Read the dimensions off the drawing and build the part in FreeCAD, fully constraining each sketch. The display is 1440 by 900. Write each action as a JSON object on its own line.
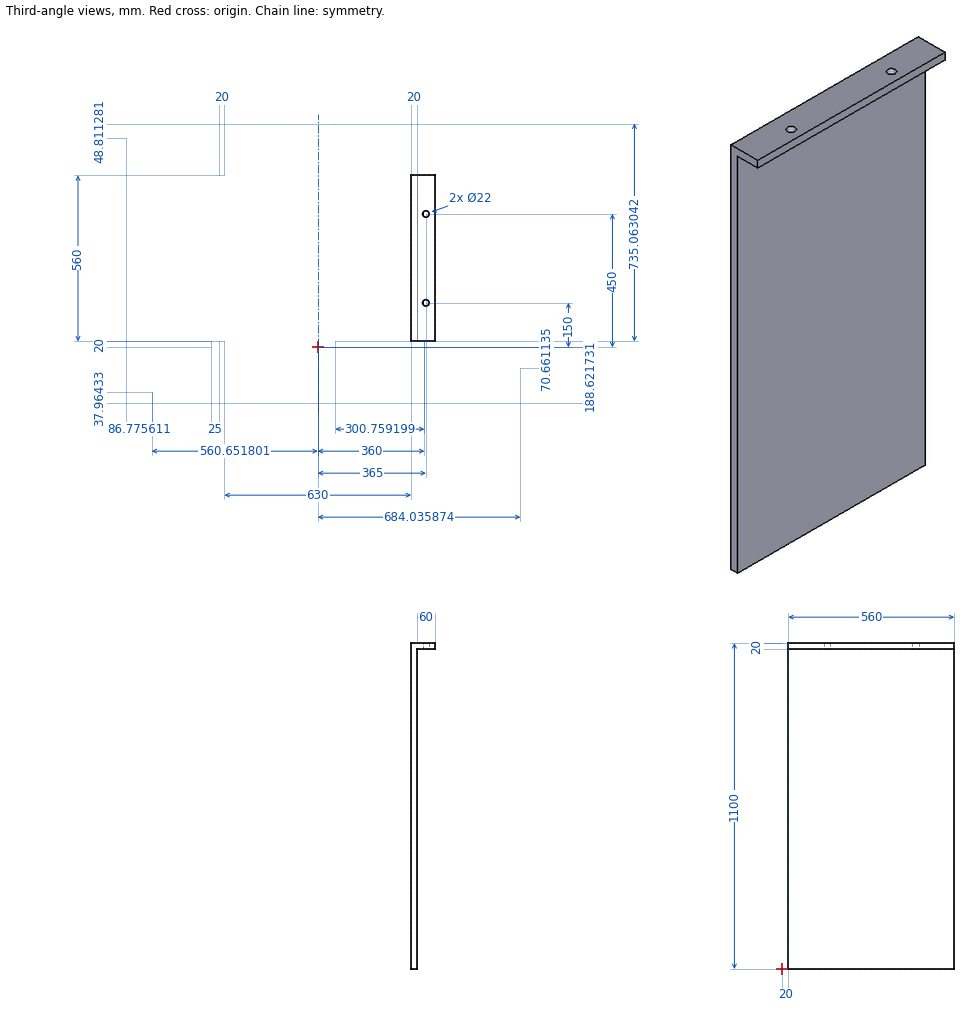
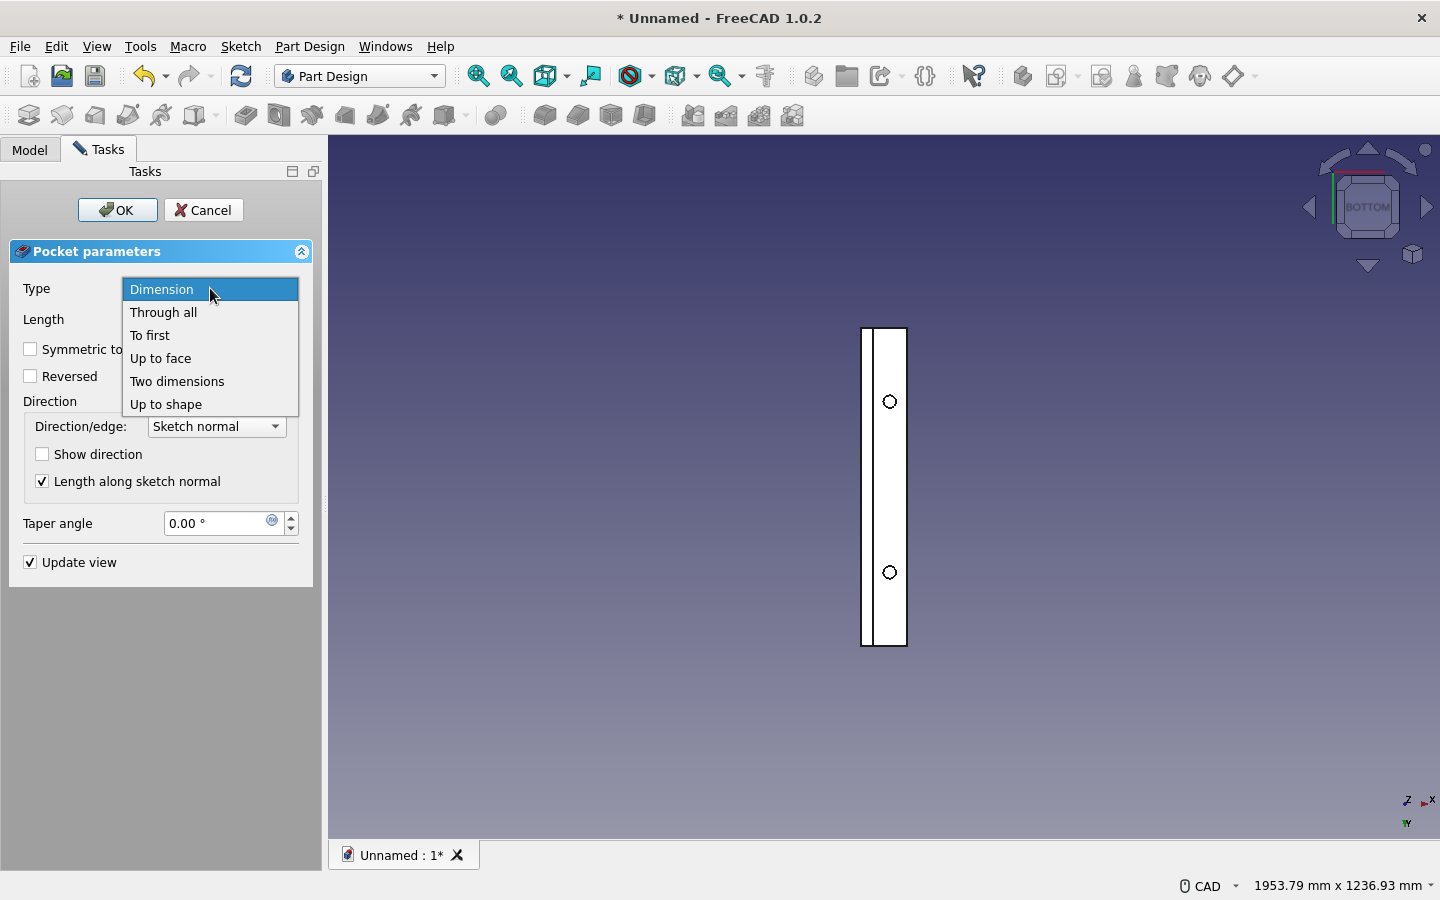
{"action": "left_click", "coordinate": [208, 312]}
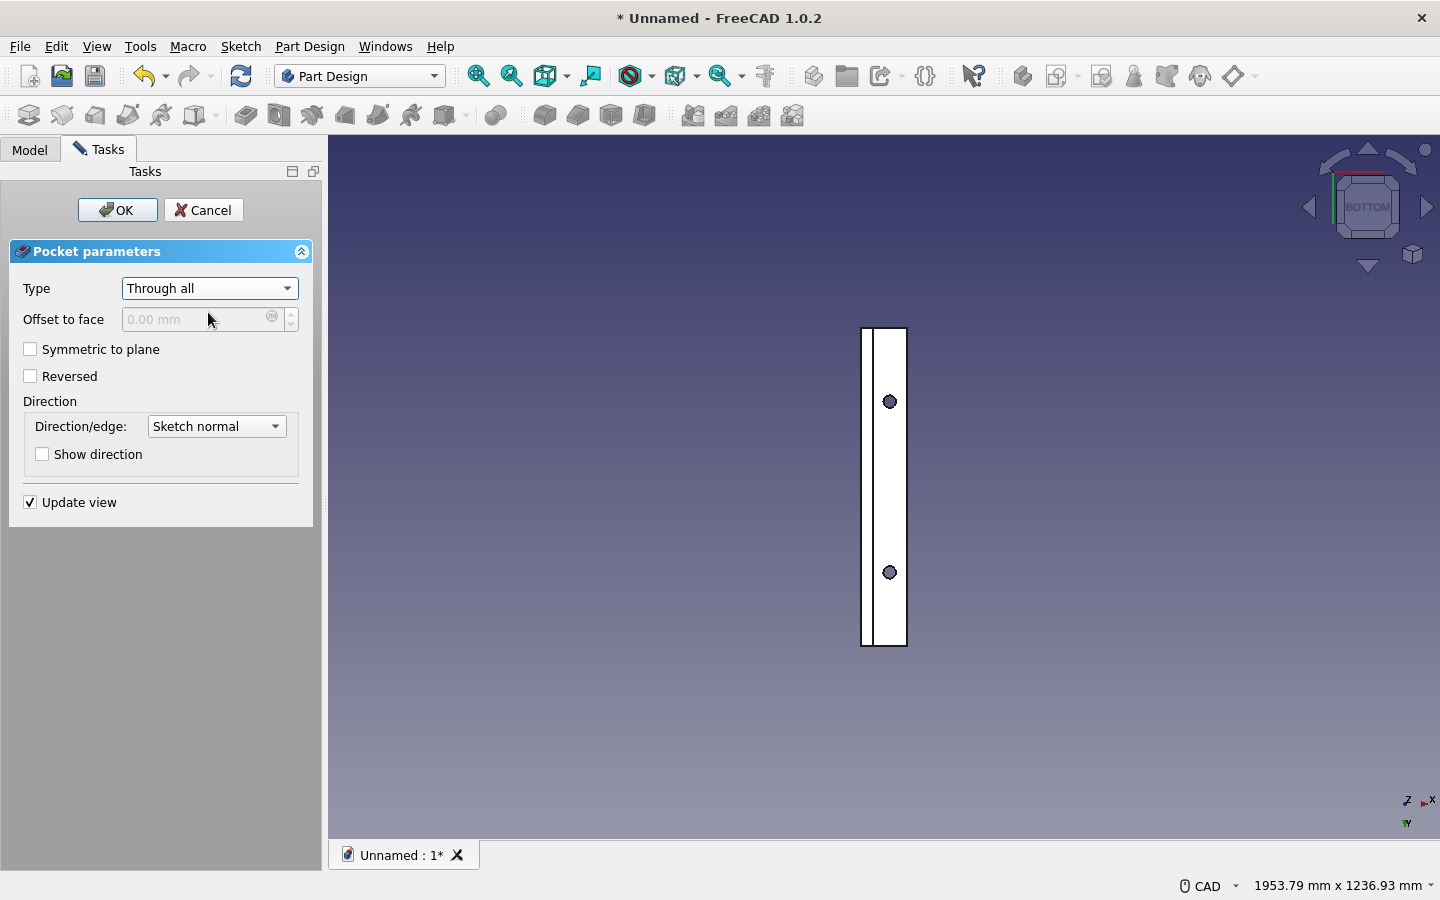
{"action": "left_click", "coordinate": [118, 210]}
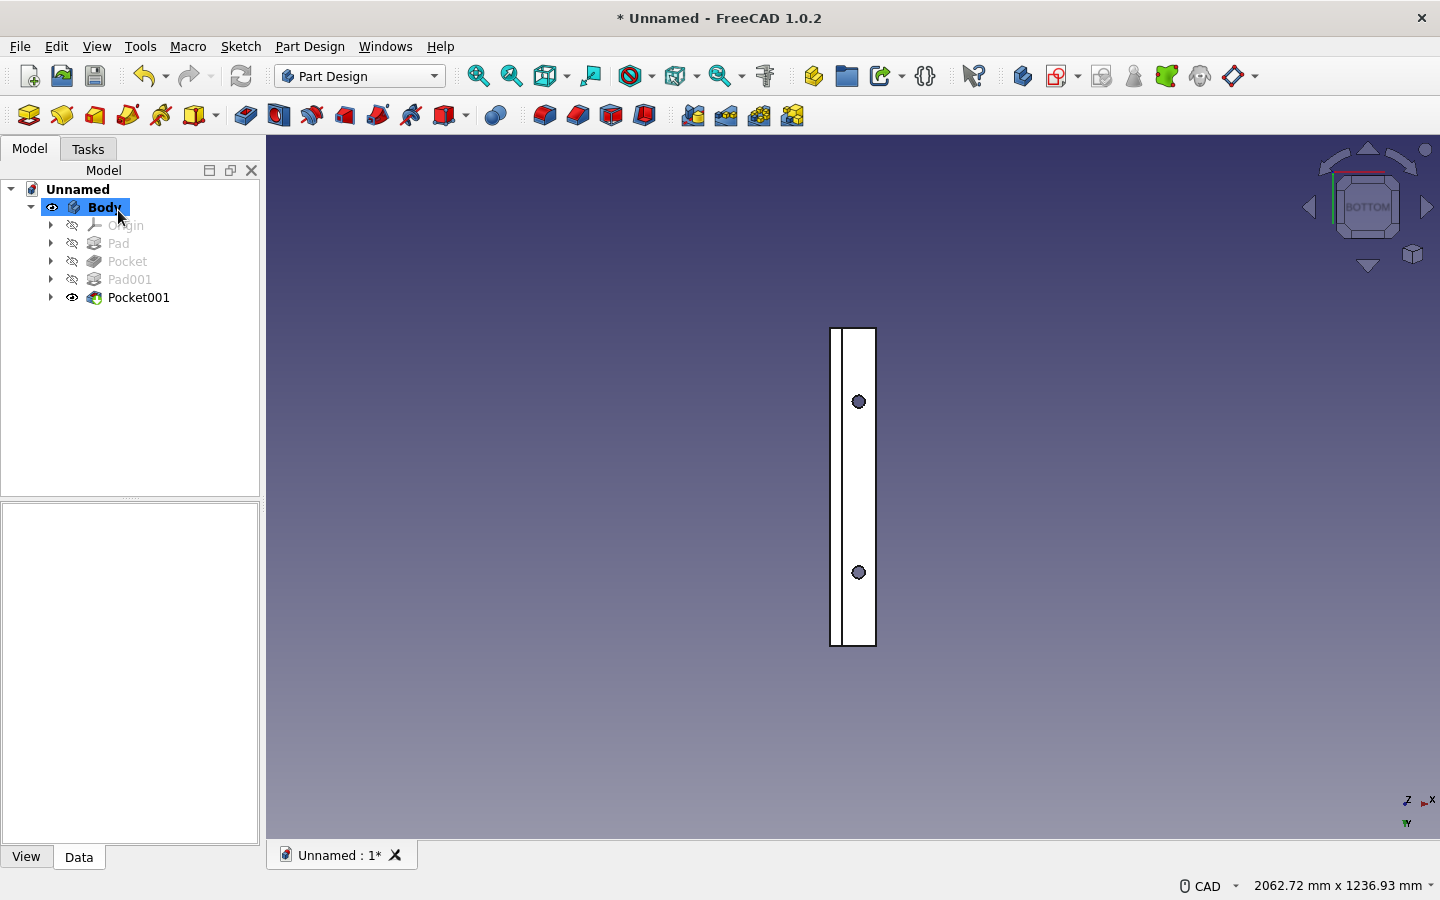
{"action": "key", "text": "0"}